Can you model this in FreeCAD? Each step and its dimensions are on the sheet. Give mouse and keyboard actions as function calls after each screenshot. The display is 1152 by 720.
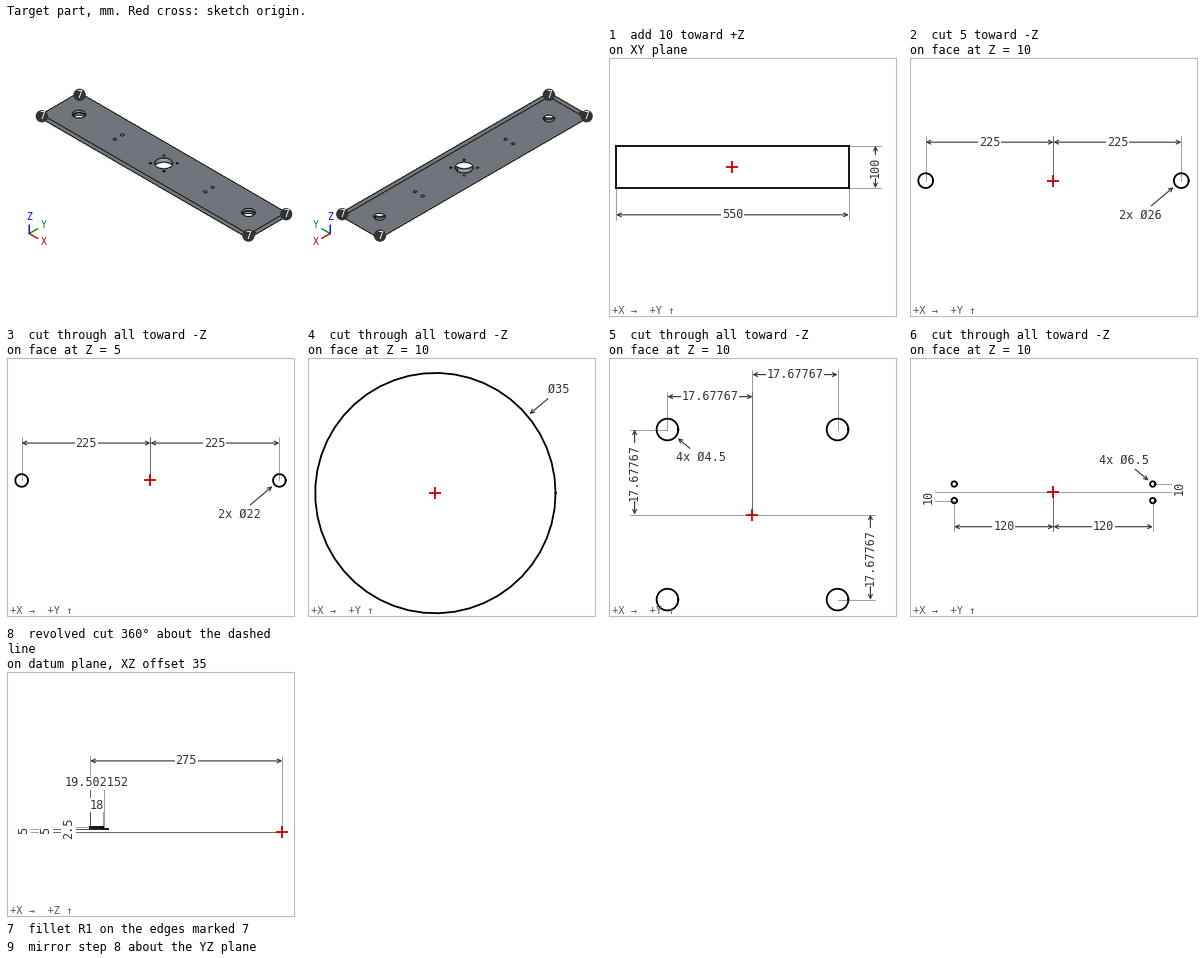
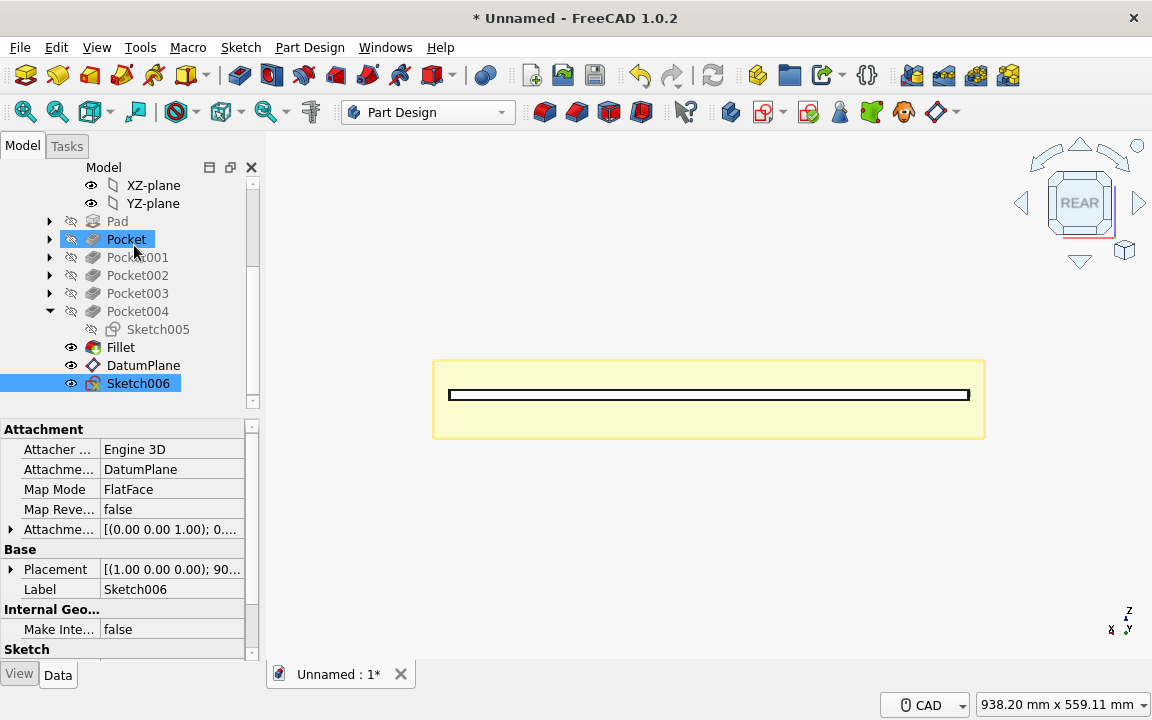
click(304, 76)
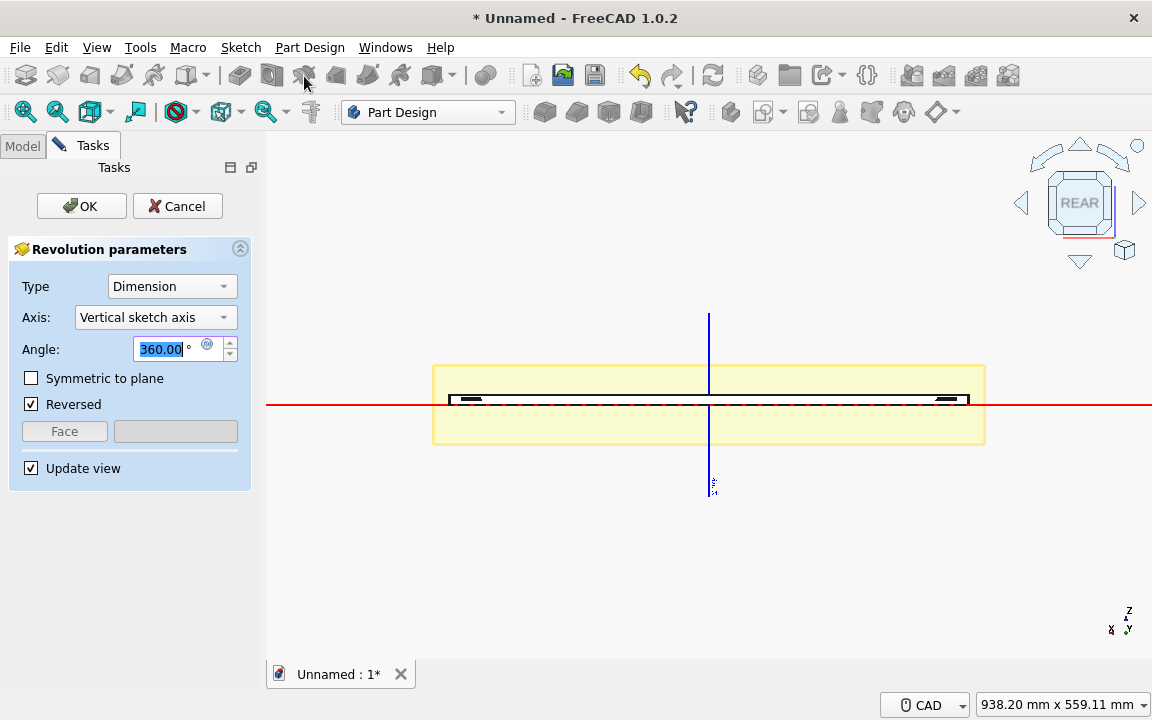
click(156, 318)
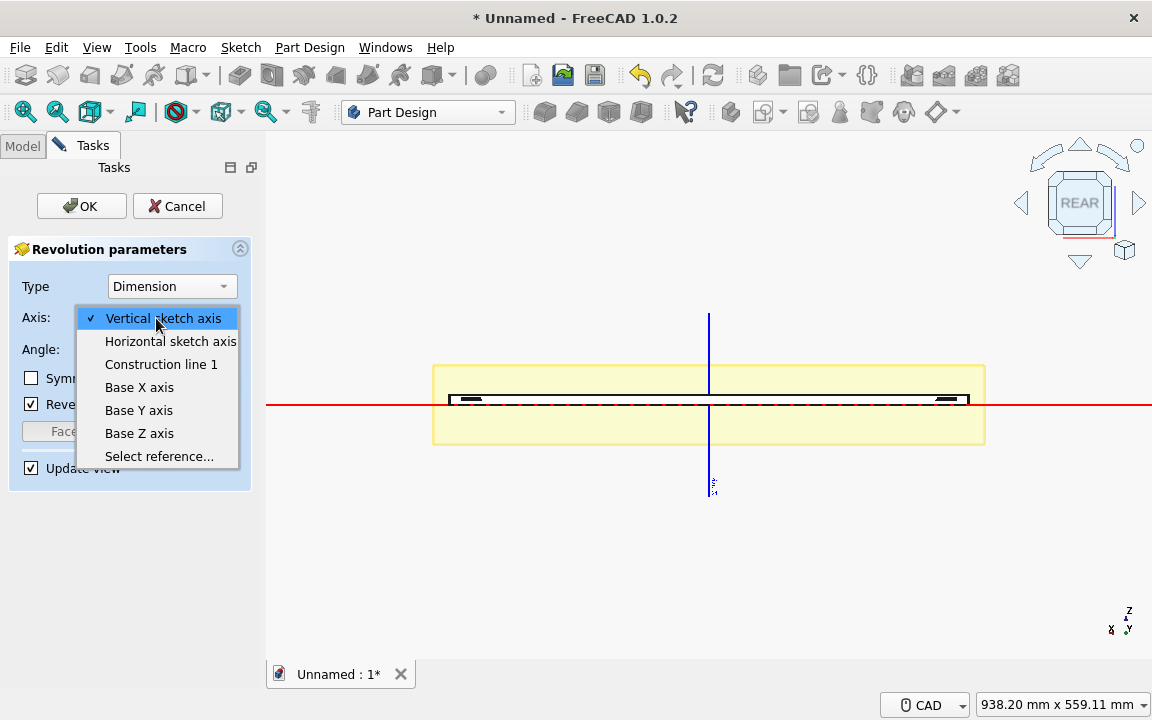
click(156, 364)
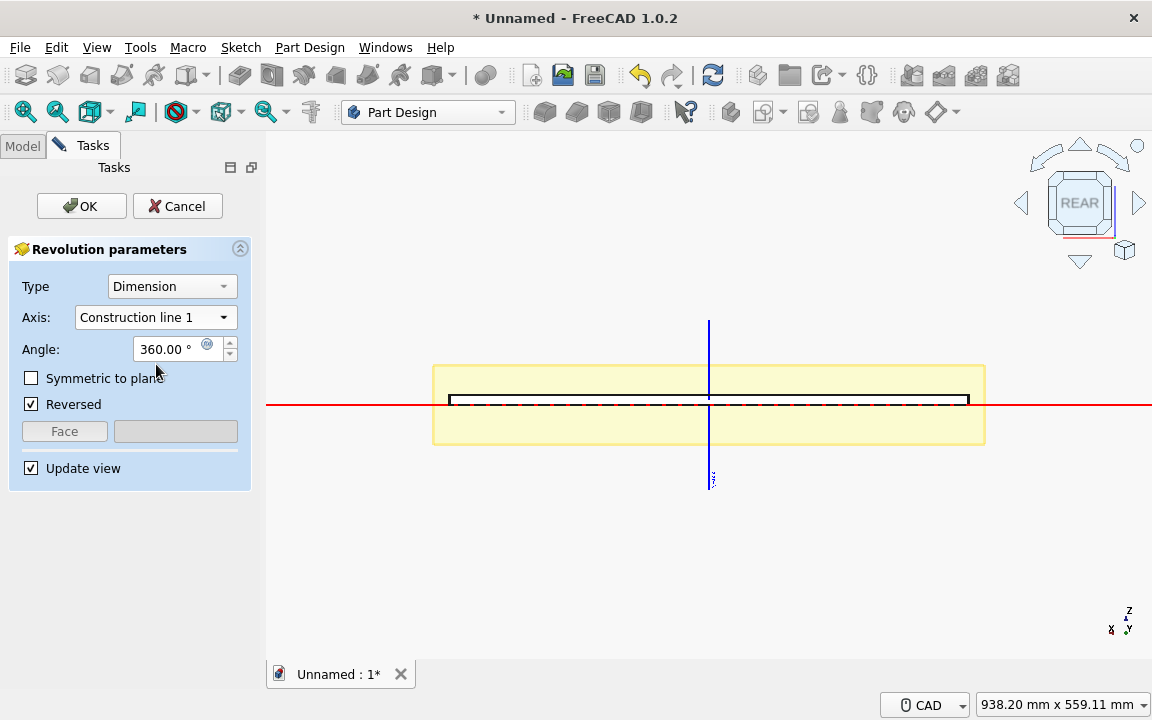
click(82, 206)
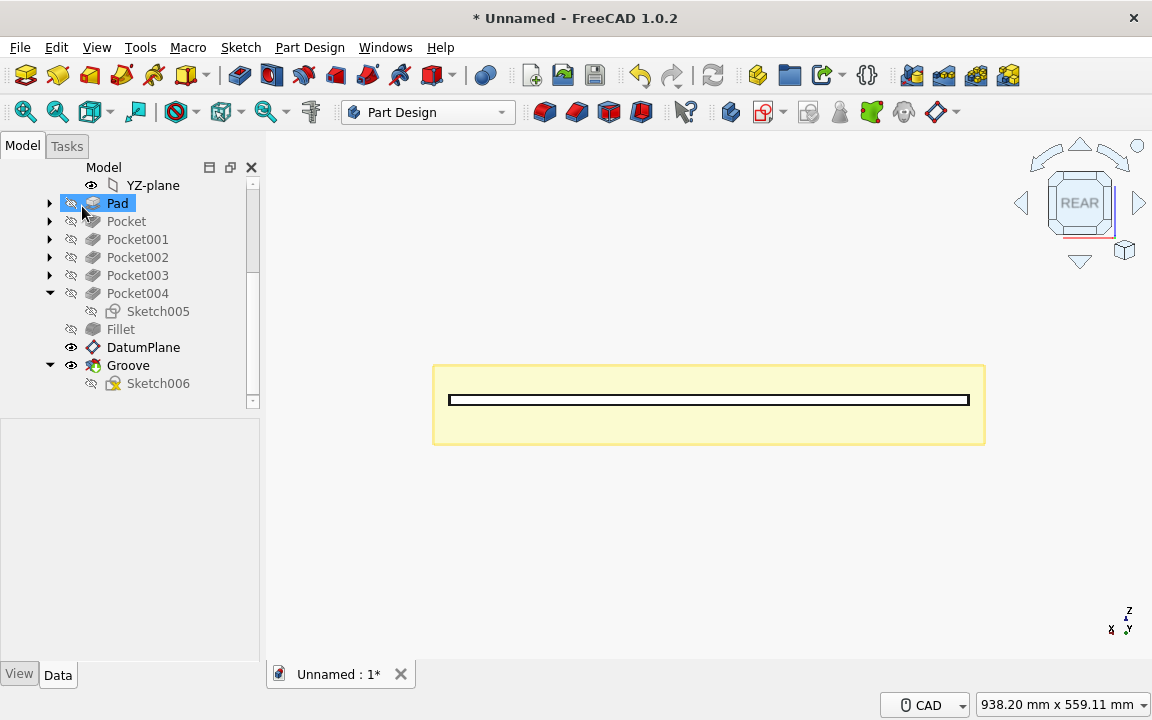
click(116, 347)
key(space)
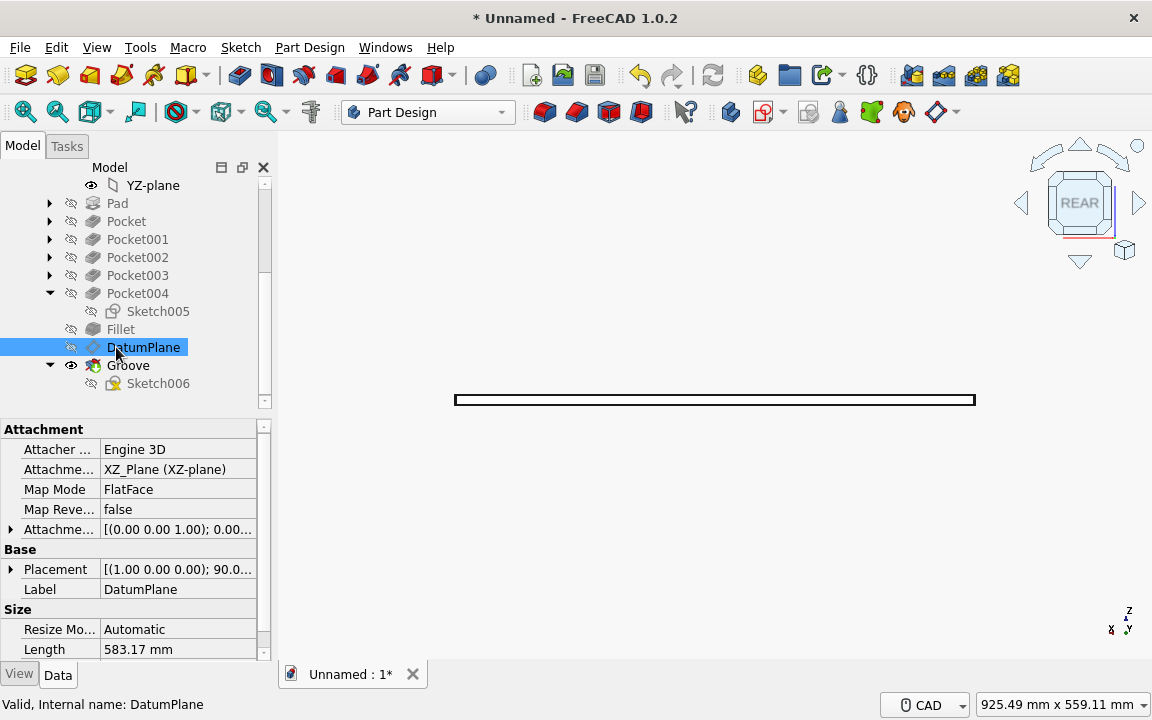
click(116, 365)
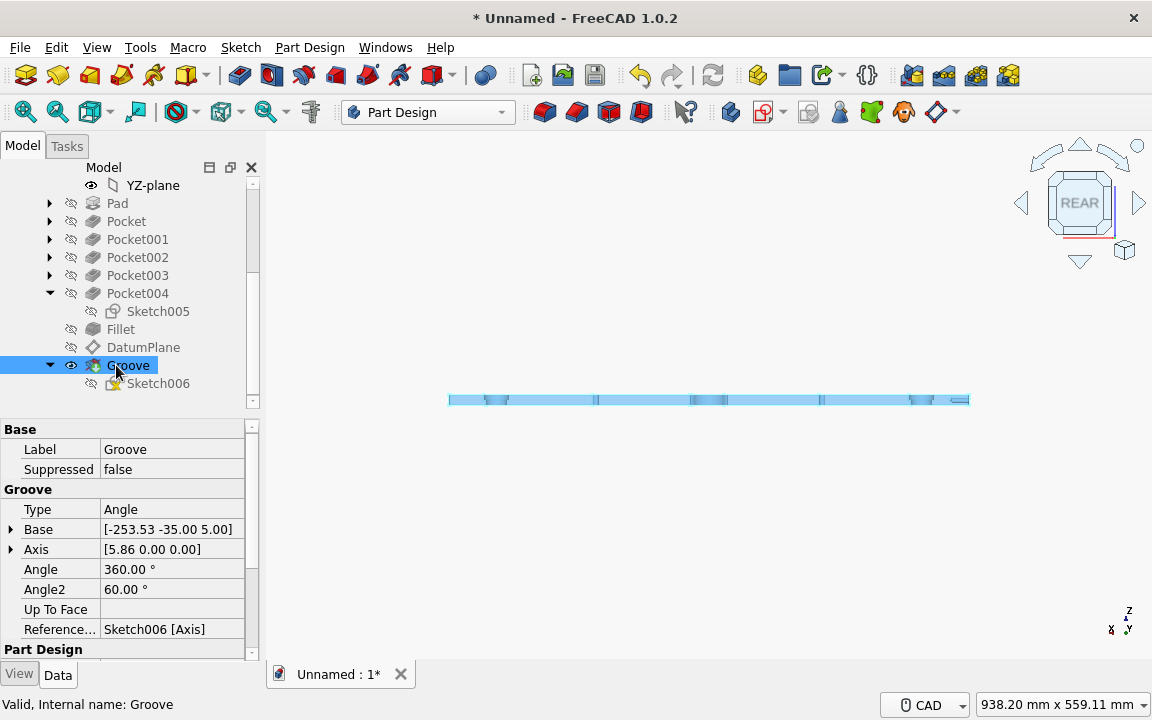
click(912, 76)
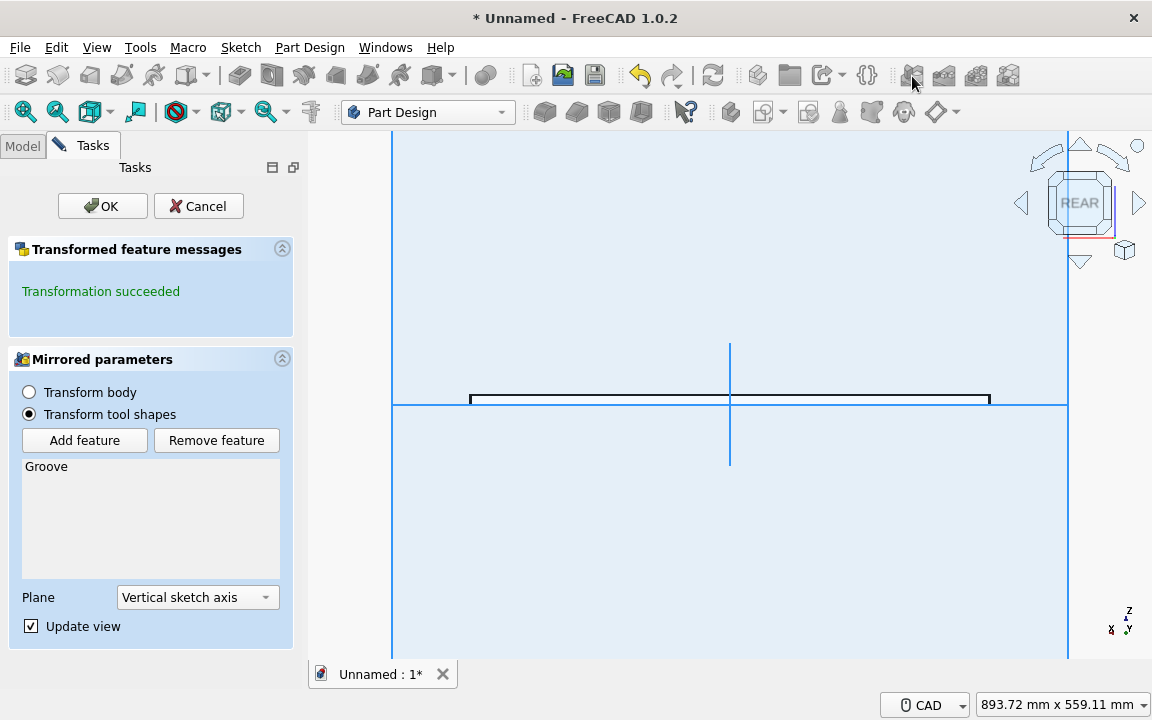
click(198, 598)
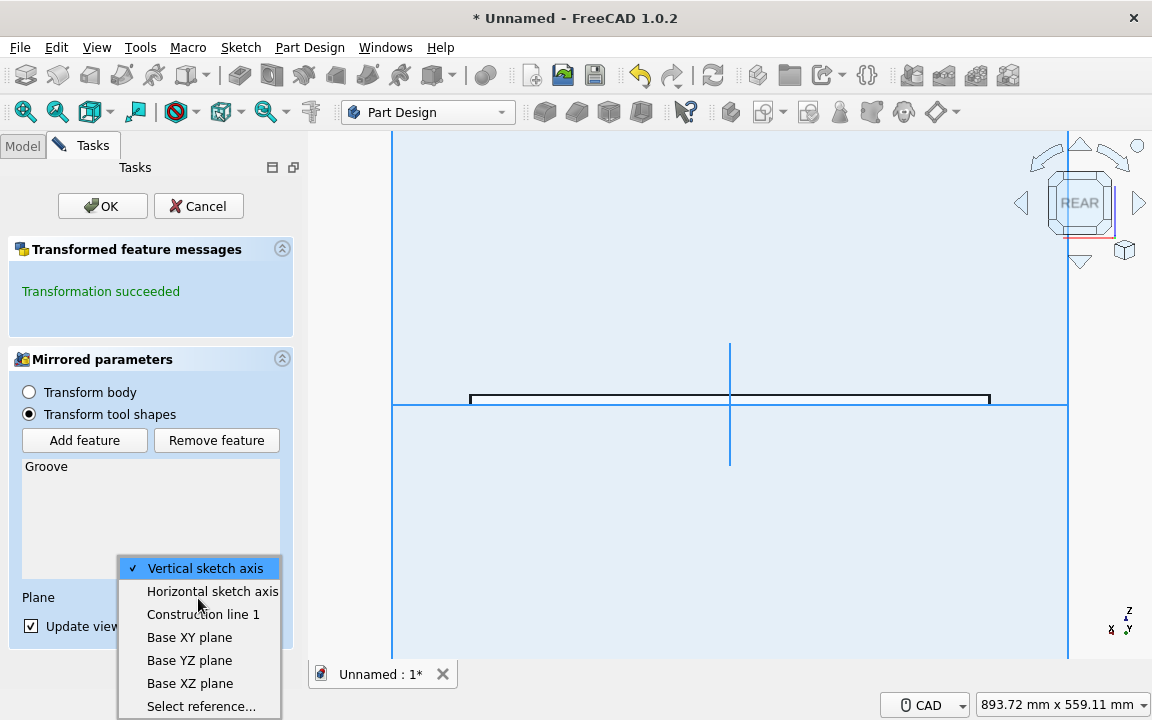
click(198, 660)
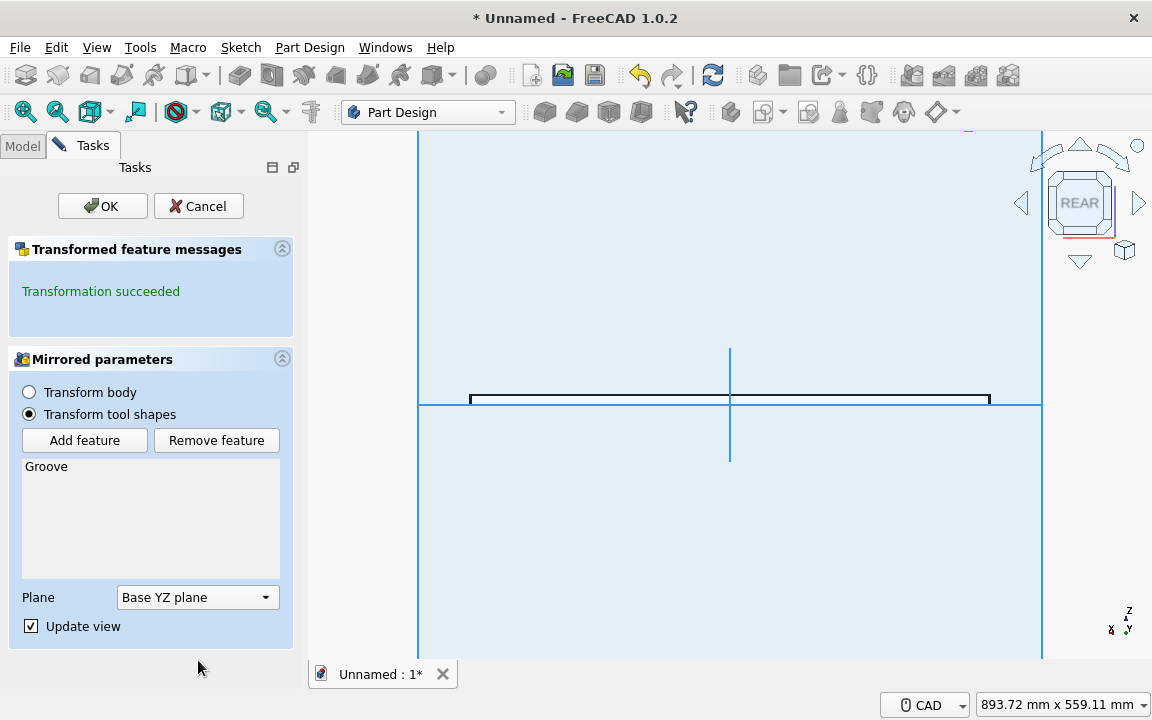
click(103, 206)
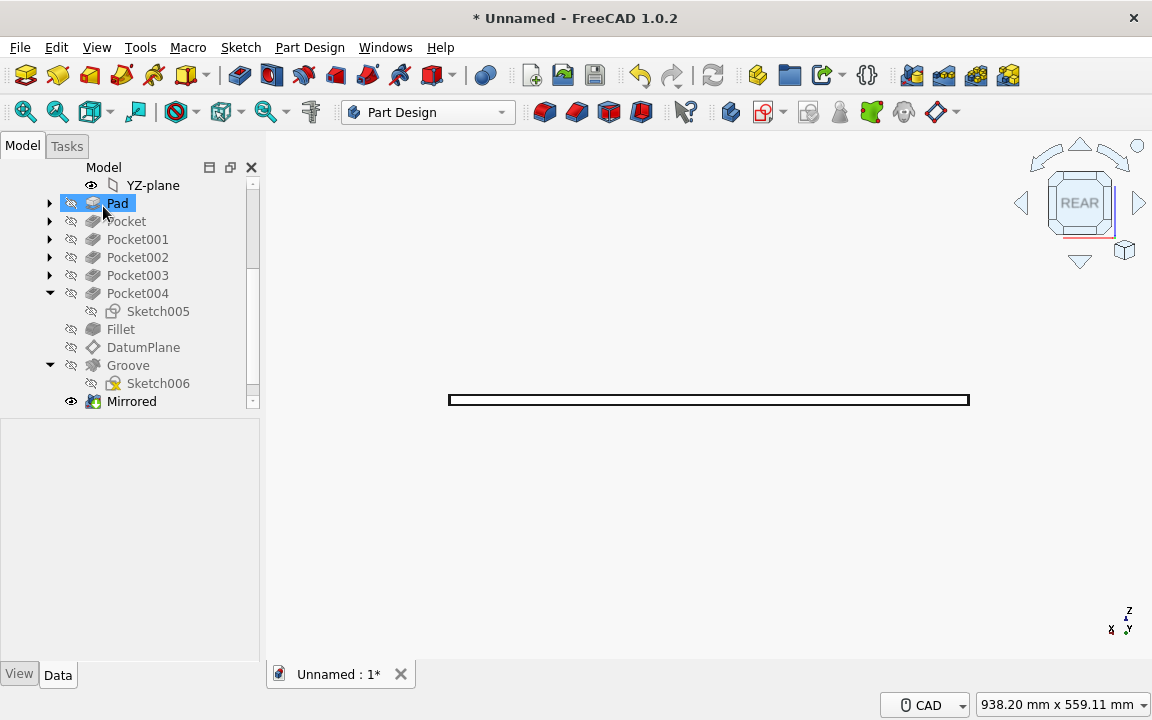
key(0)